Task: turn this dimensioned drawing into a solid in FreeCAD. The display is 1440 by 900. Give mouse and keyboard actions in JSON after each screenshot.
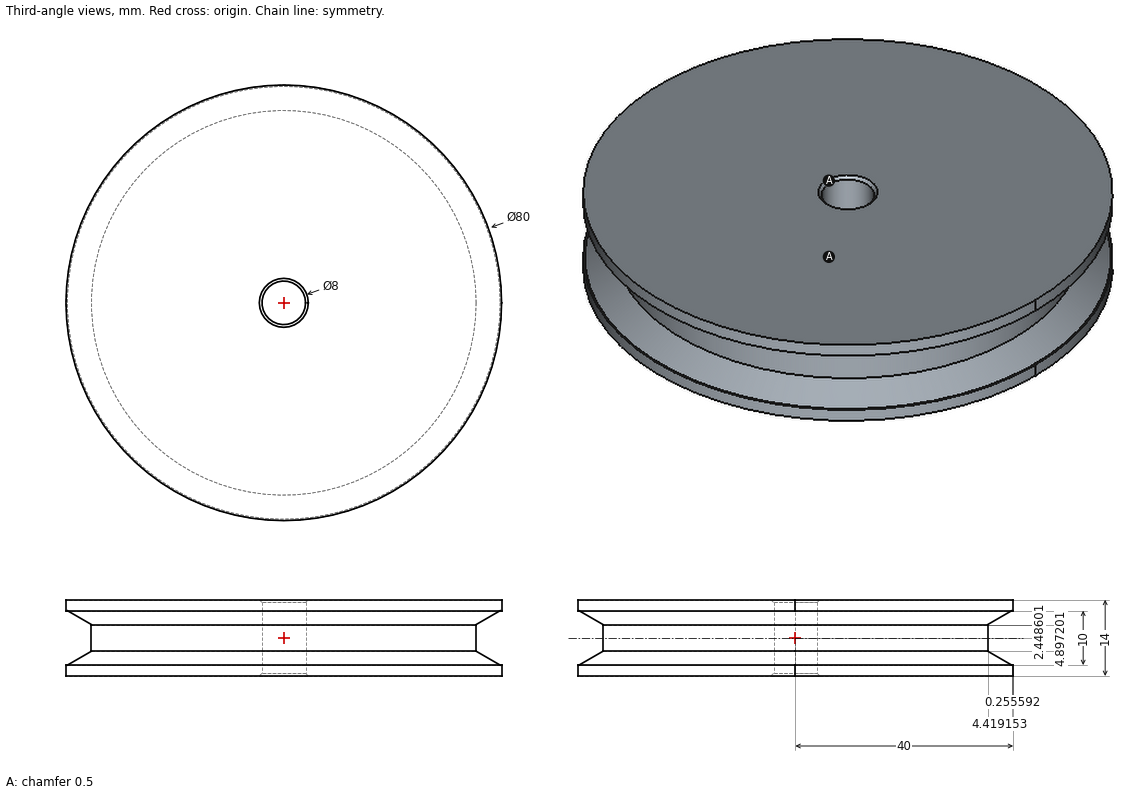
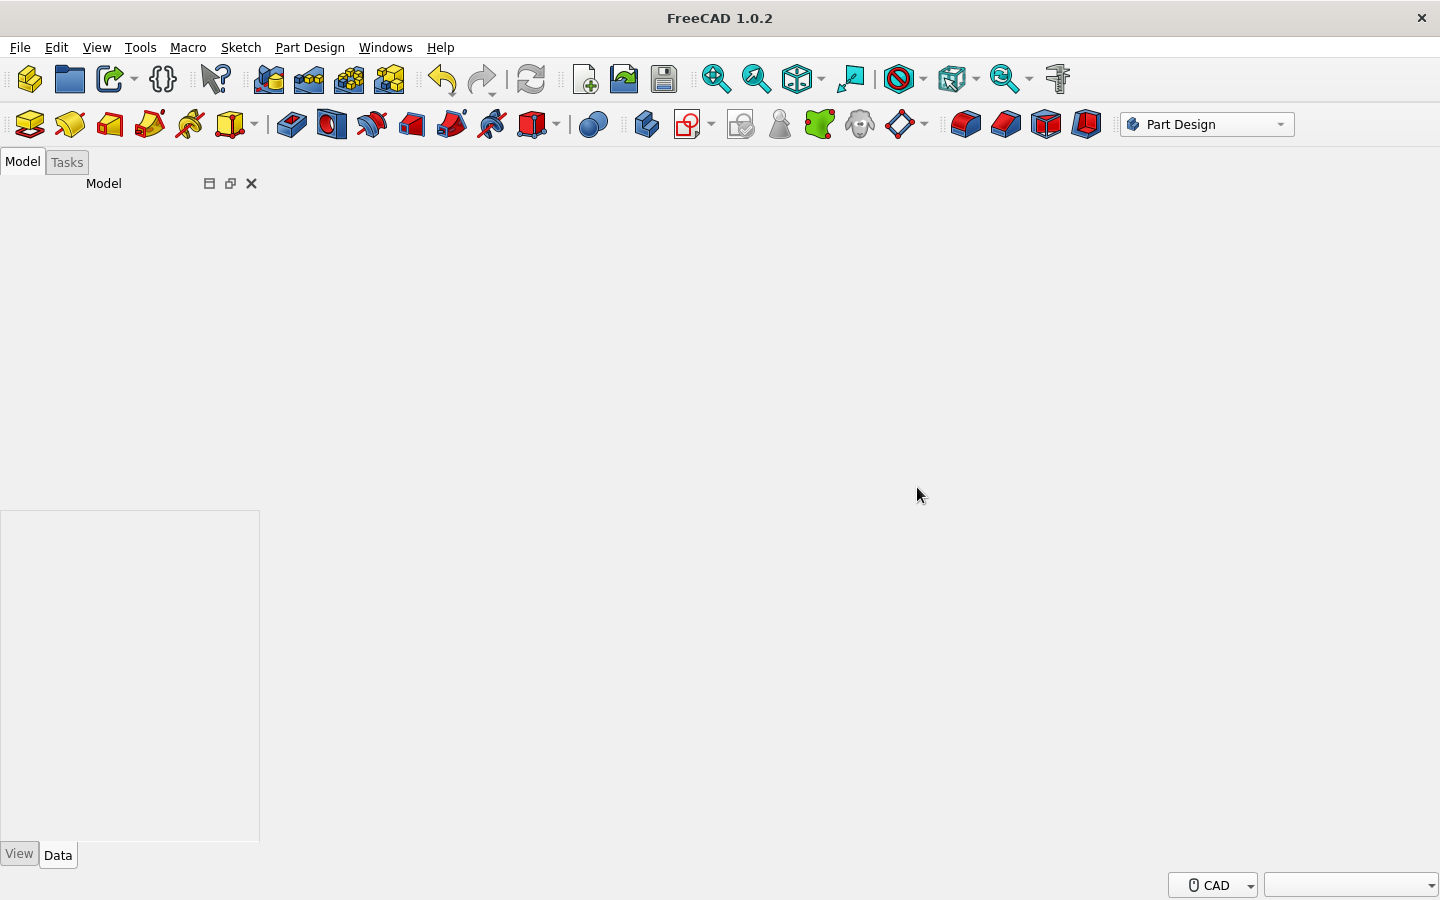
{"action": "left_click", "coordinate": [584, 80]}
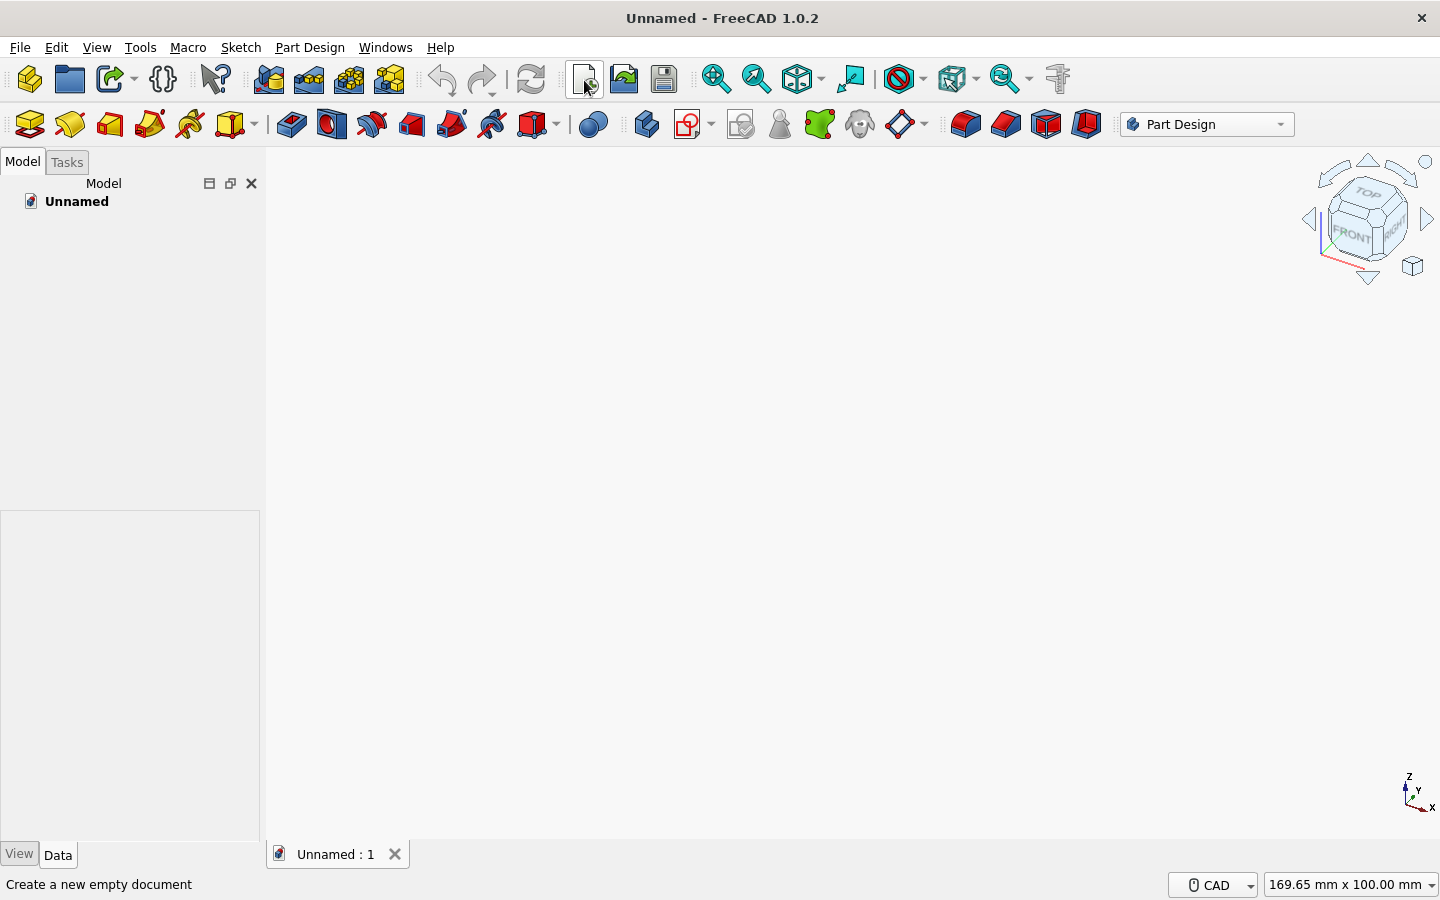
{"action": "left_click", "coordinate": [688, 124]}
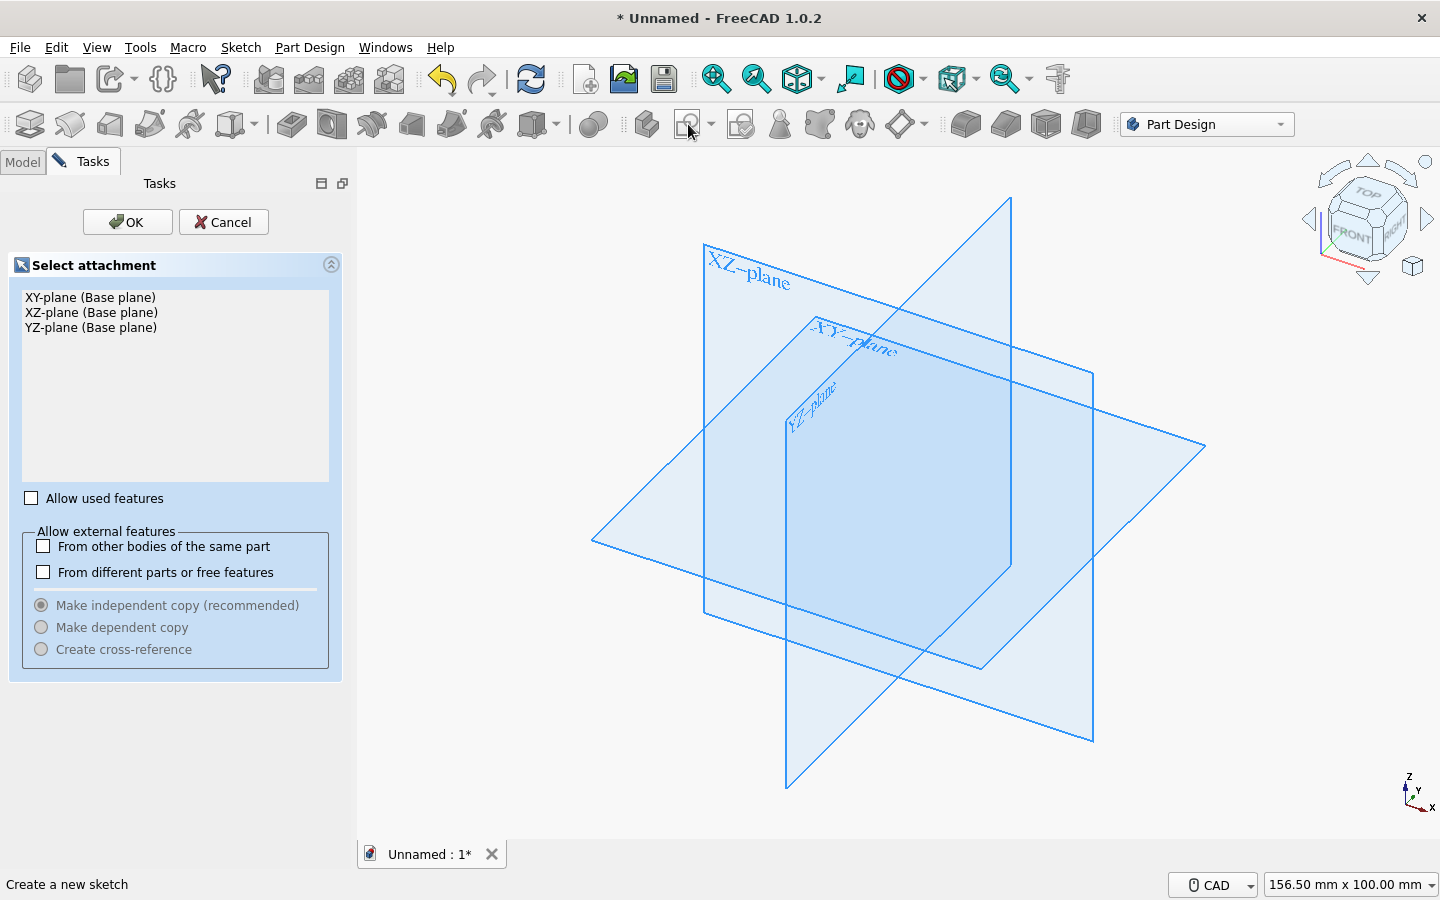
{"action": "left_click", "coordinate": [82, 298]}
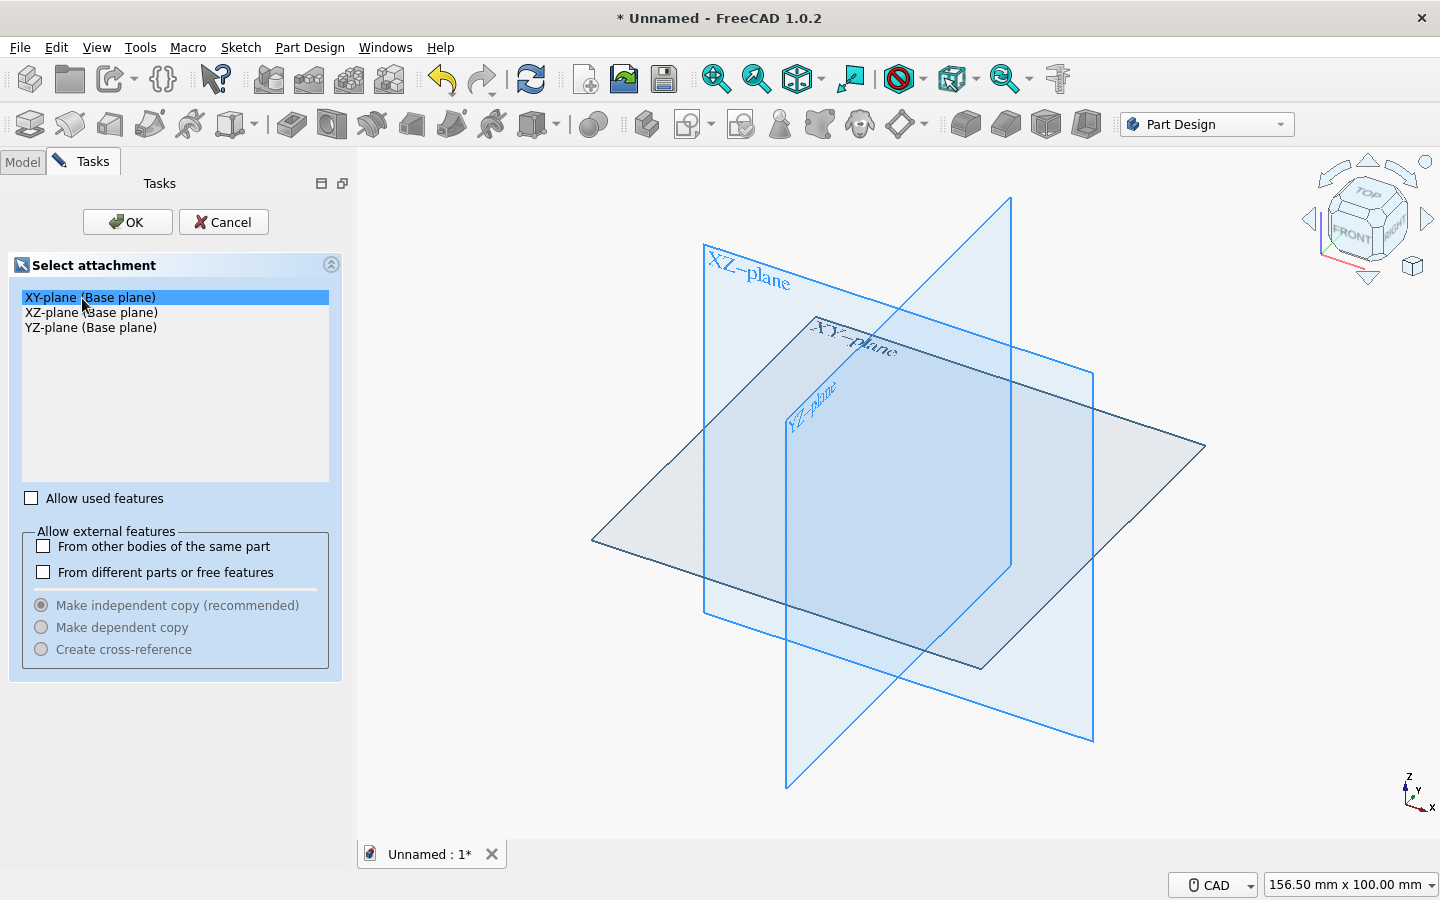
{"action": "left_click", "coordinate": [128, 222]}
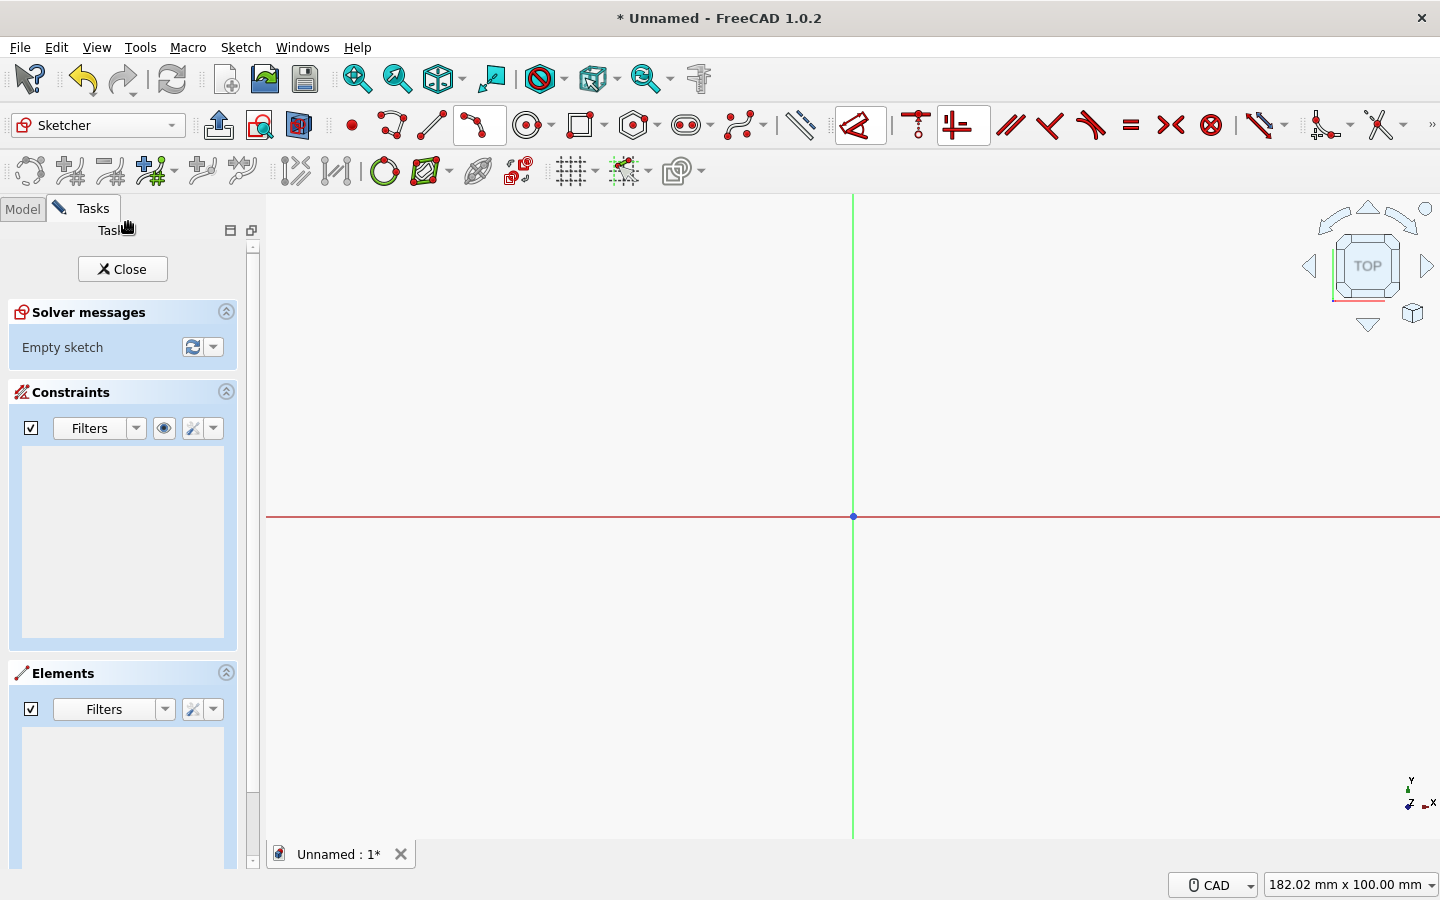
{"action": "left_click", "coordinate": [528, 126]}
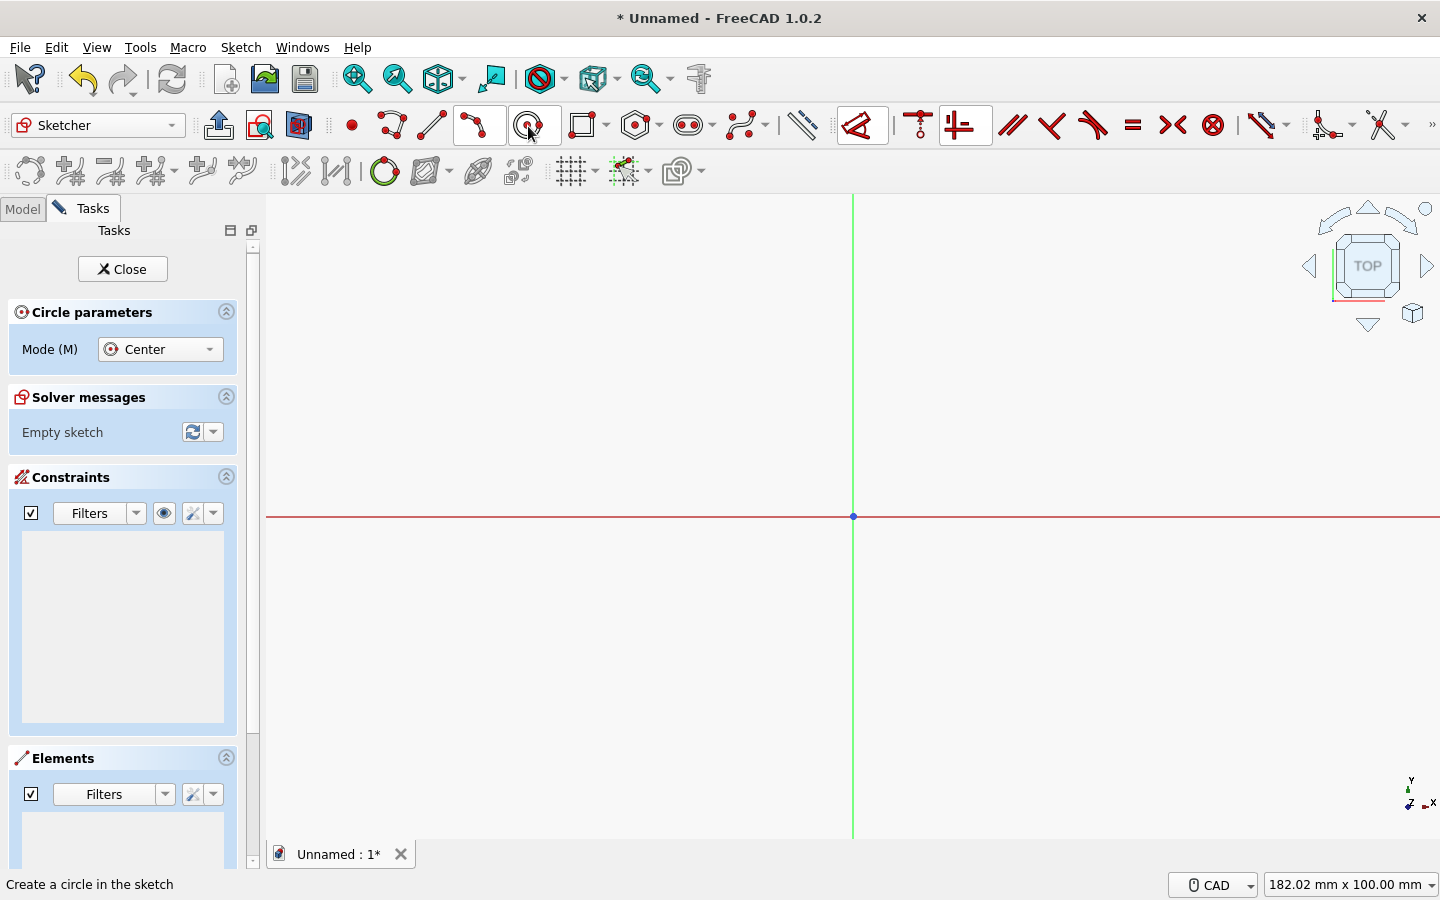
{"action": "left_click", "coordinate": [853, 516]}
{"action": "mouse_move", "coordinate": [1035, 334]}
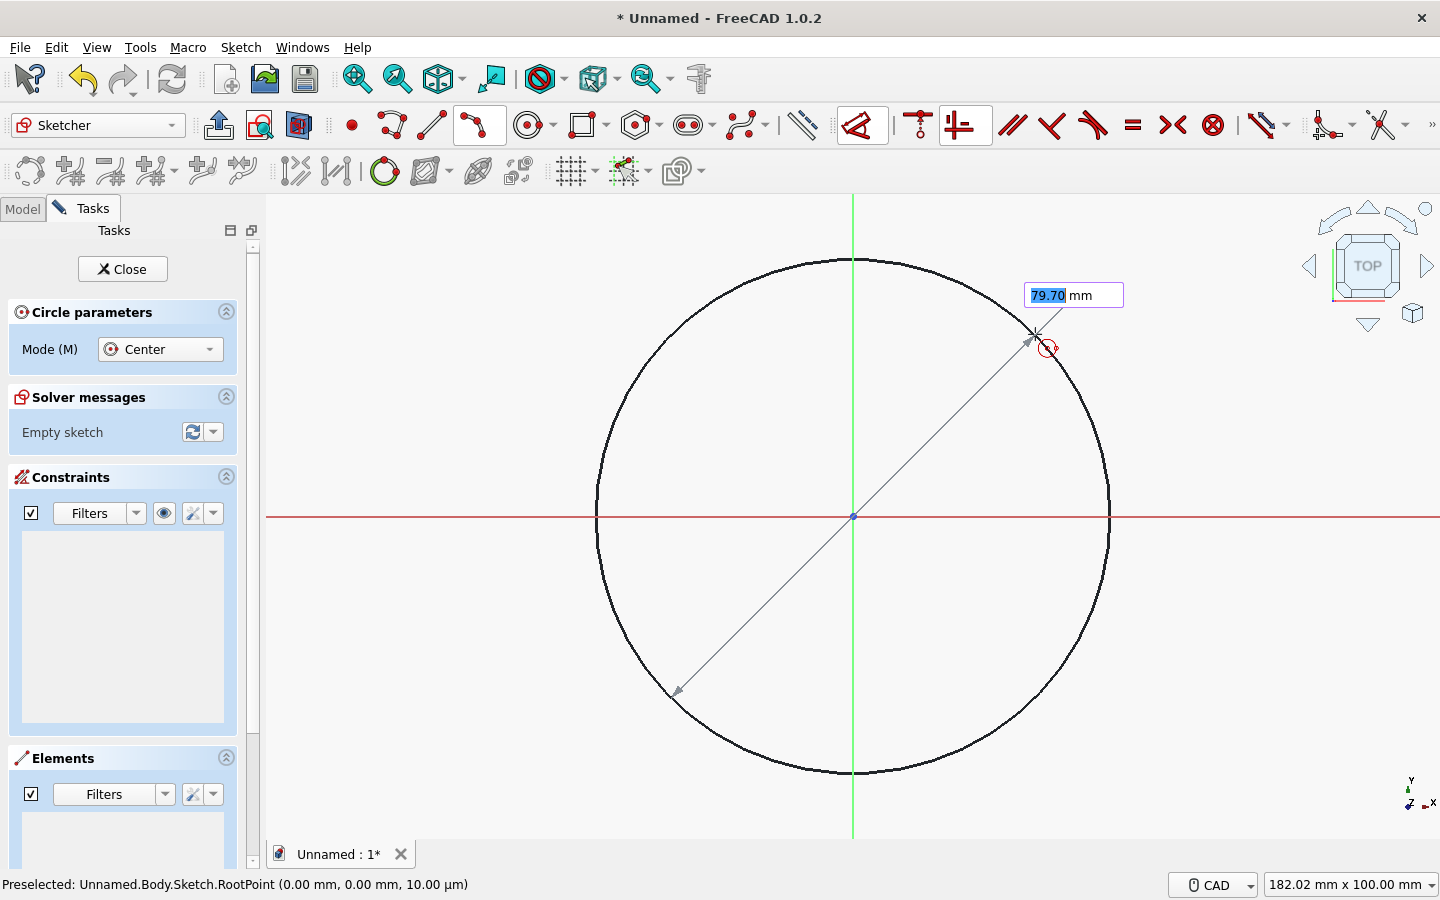
{"action": "type", "text": "80"}
{"action": "key", "text": "Return"}